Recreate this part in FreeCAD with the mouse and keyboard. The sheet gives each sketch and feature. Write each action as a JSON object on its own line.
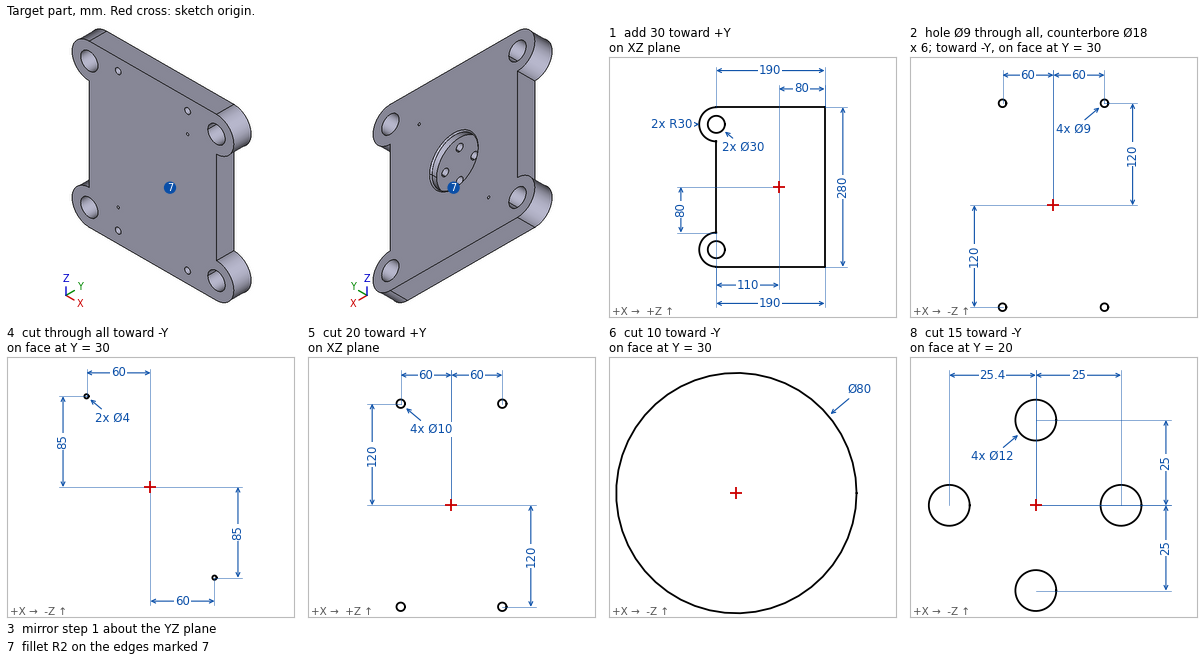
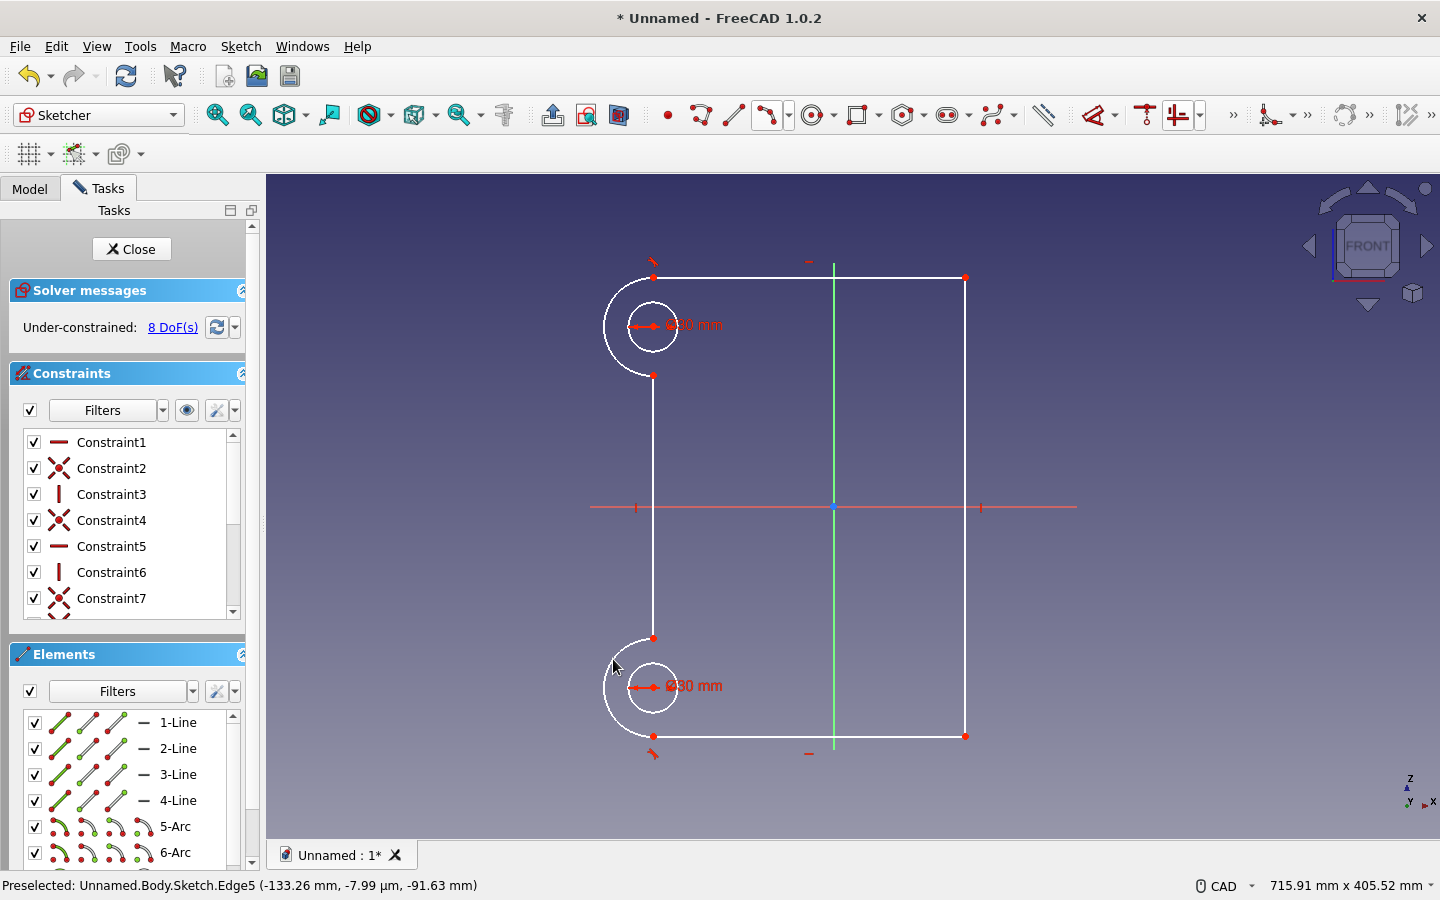
{"action": "left_click", "coordinate": [613, 659]}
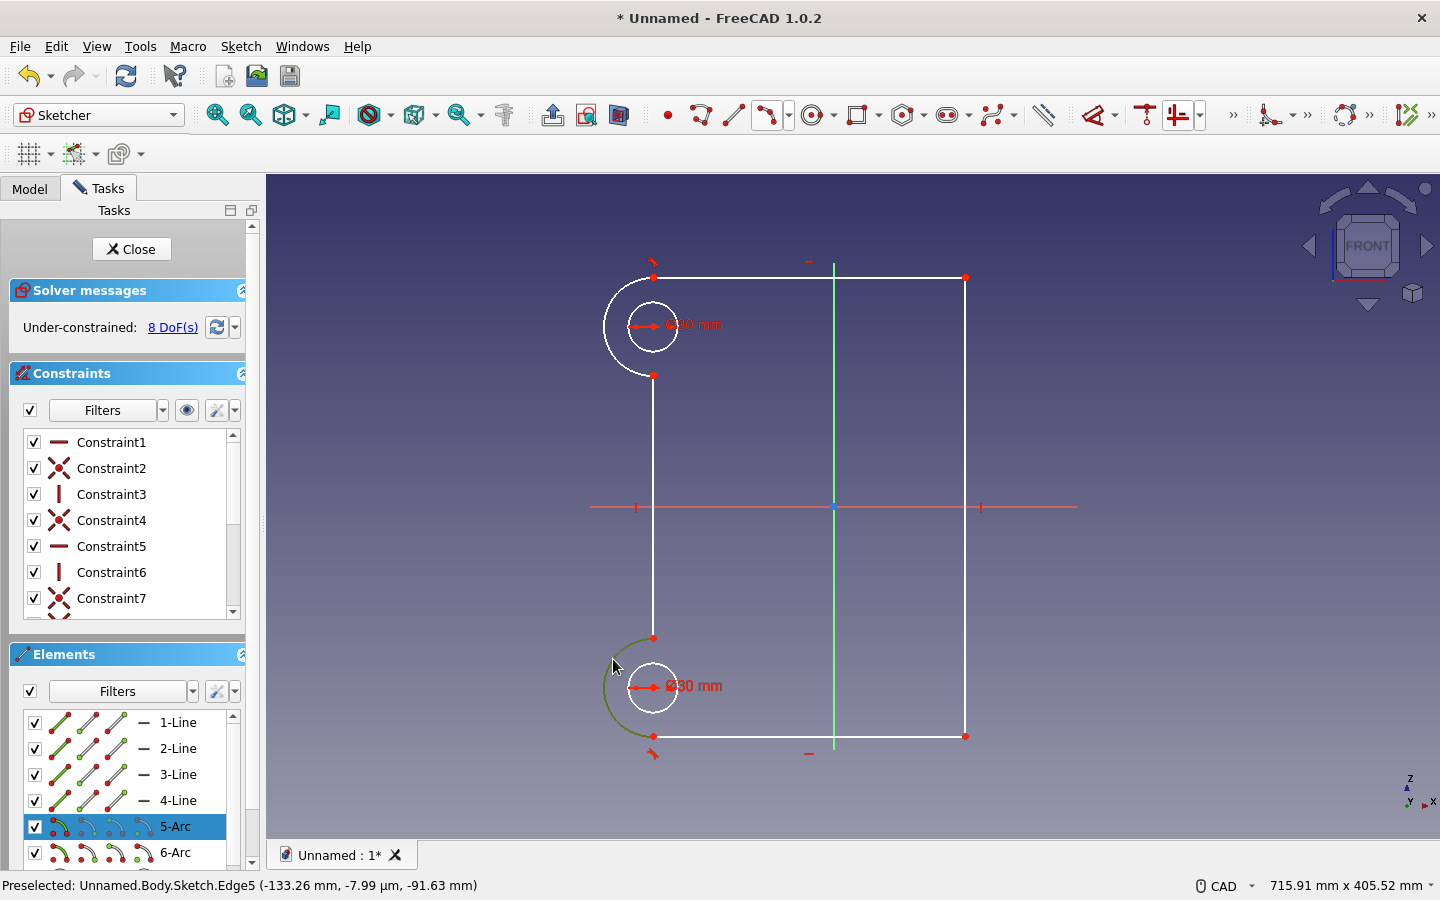
{"action": "left_click", "coordinate": [613, 298]}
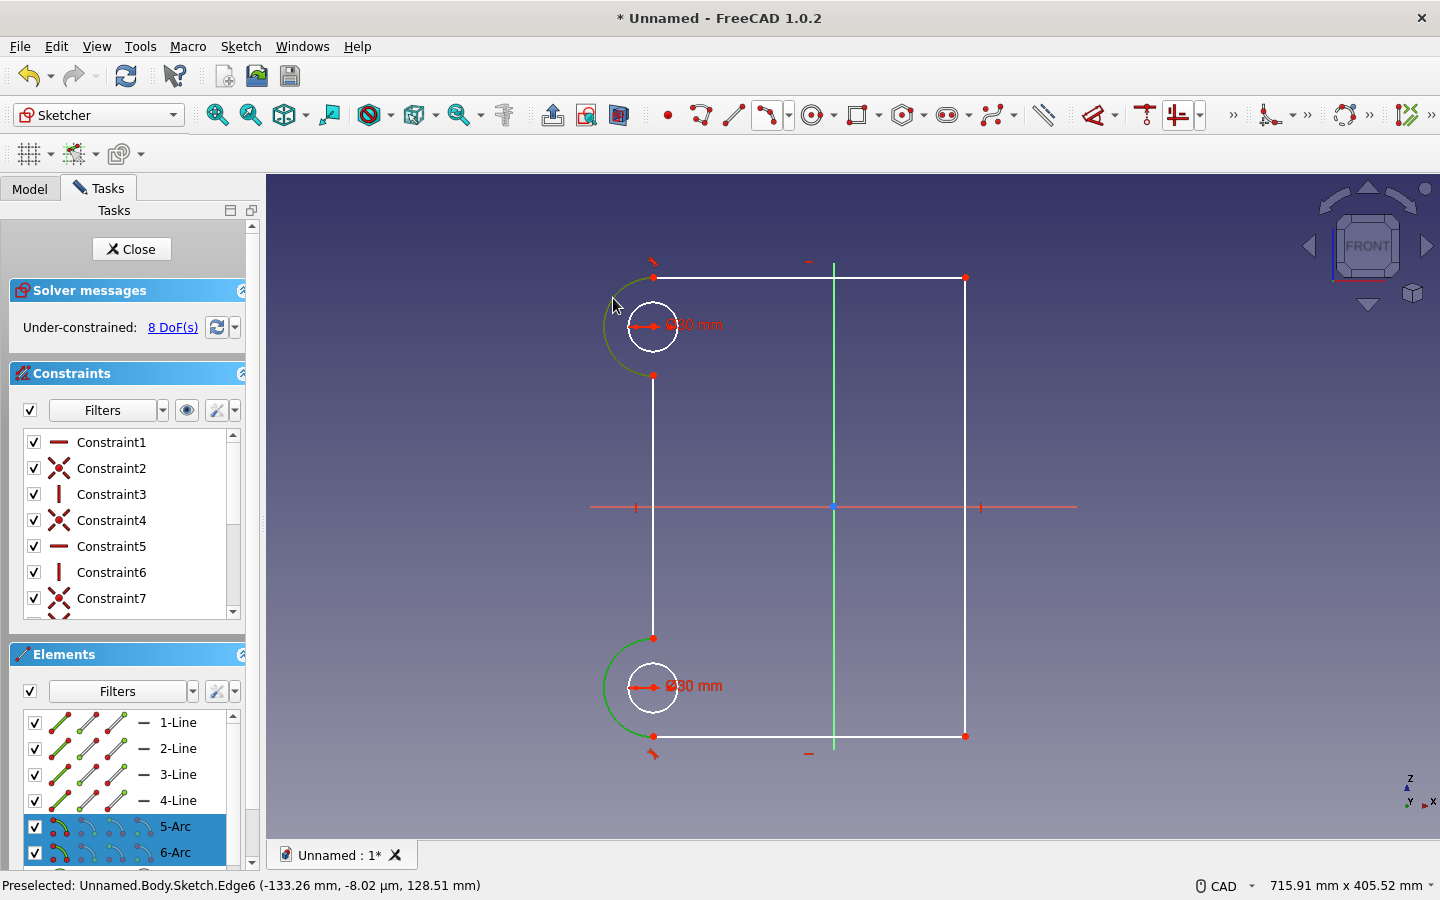
{"action": "key", "text": "e"}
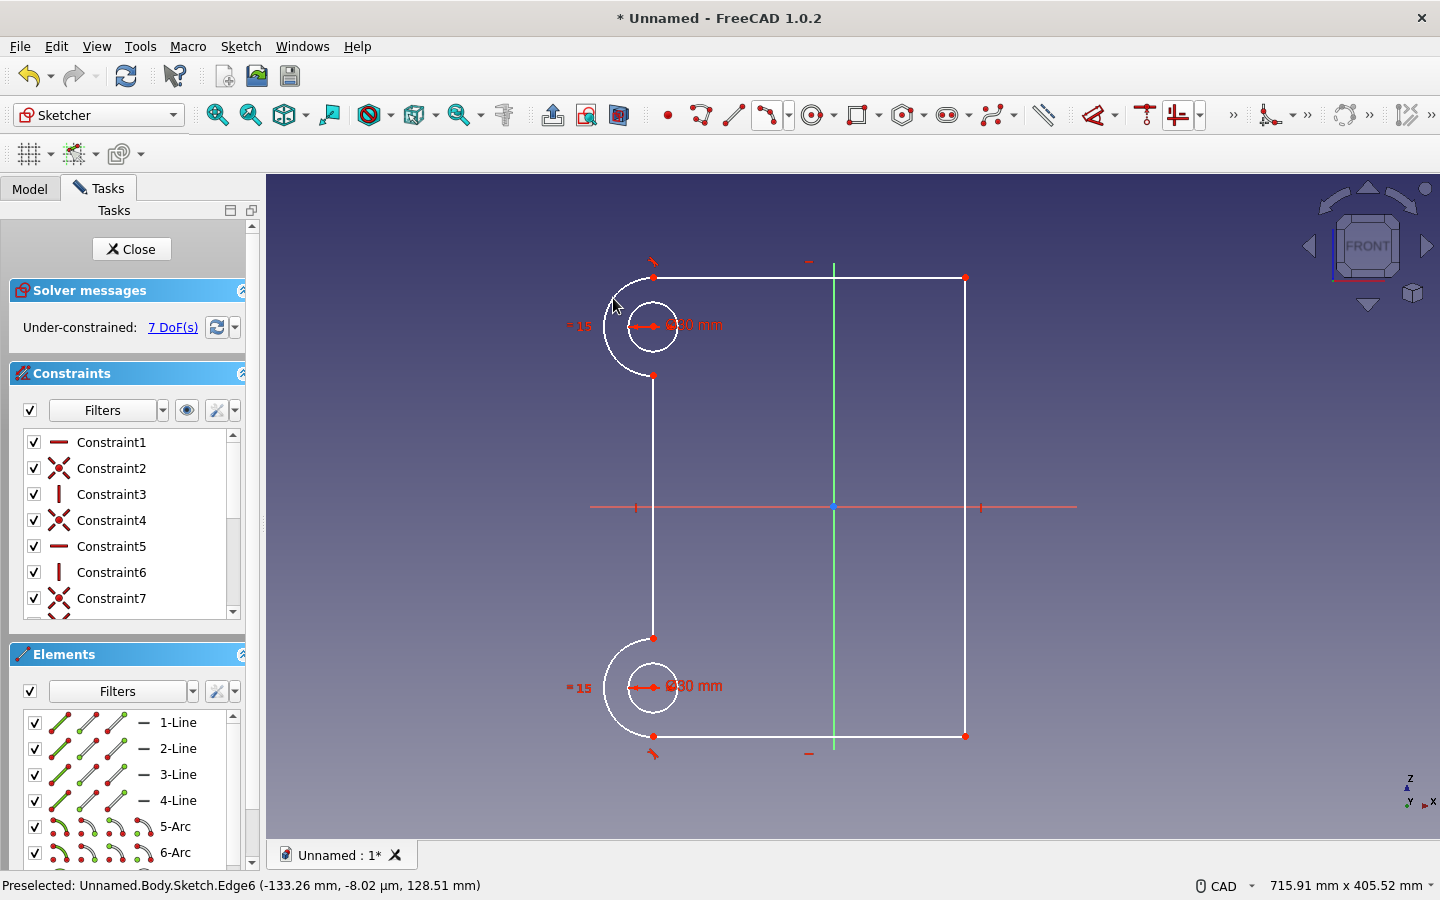
{"action": "left_click", "coordinate": [1092, 116]}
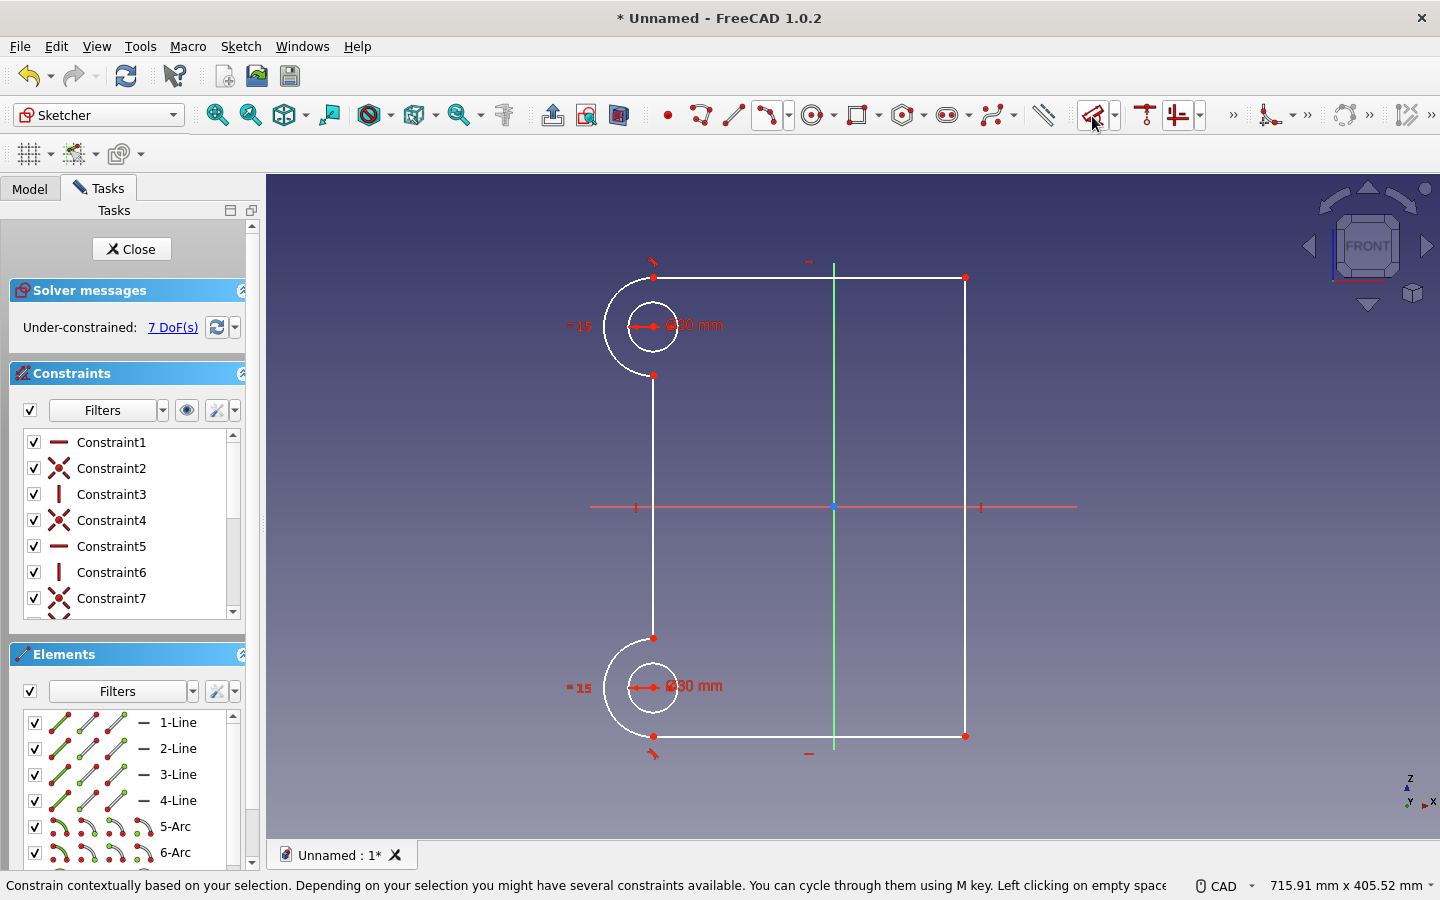
{"action": "left_click", "coordinate": [613, 659]}
{"action": "left_click", "coordinate": [587, 640]}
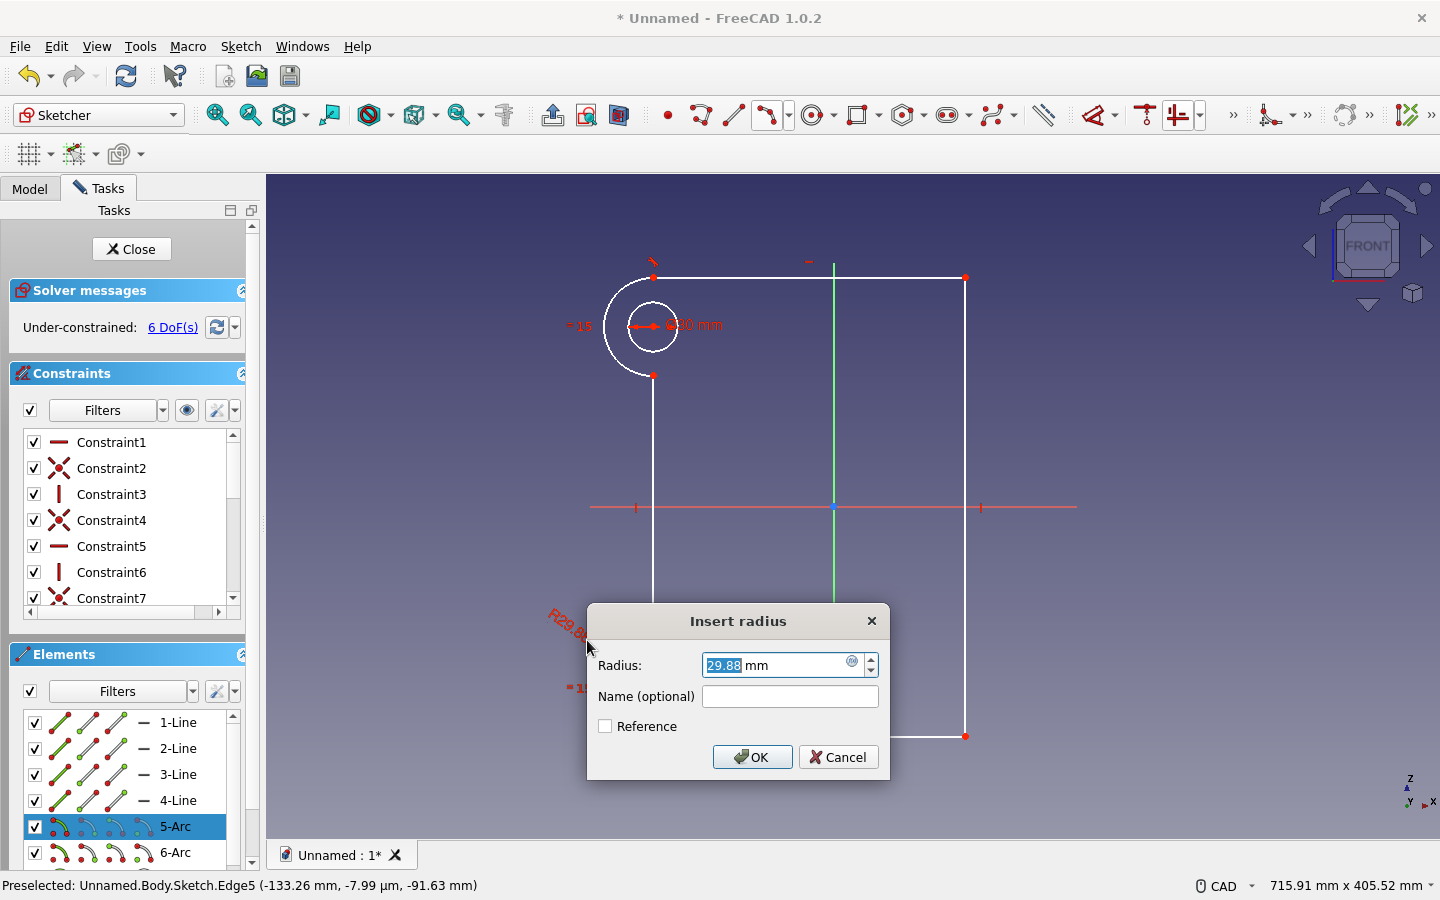
{"action": "type", "text": "30"}
{"action": "key", "text": "Return"}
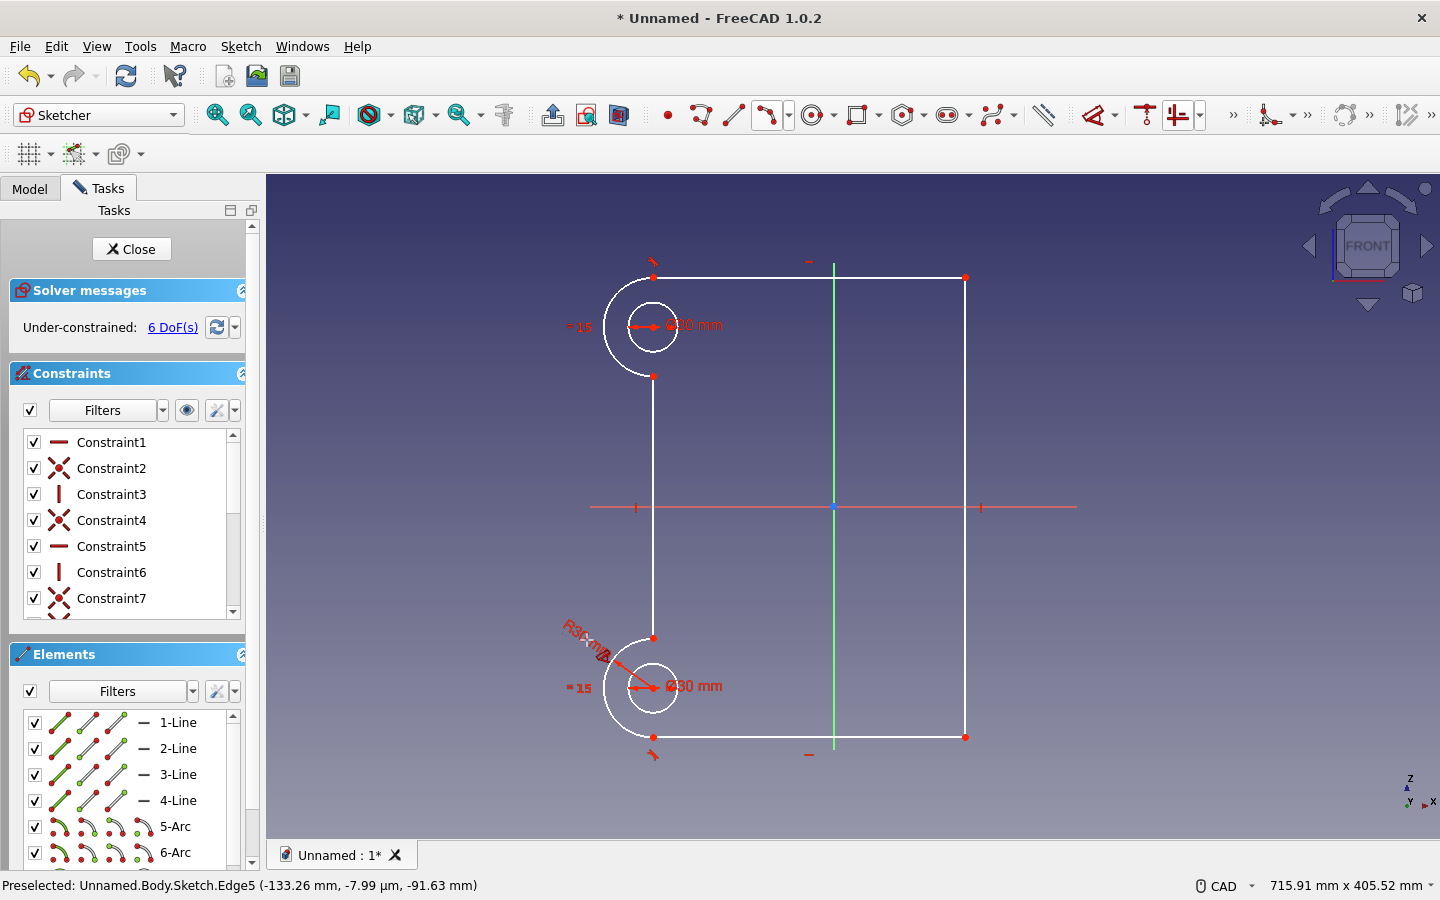
{"action": "left_click", "coordinate": [747, 278]}
{"action": "left_click", "coordinate": [809, 244]}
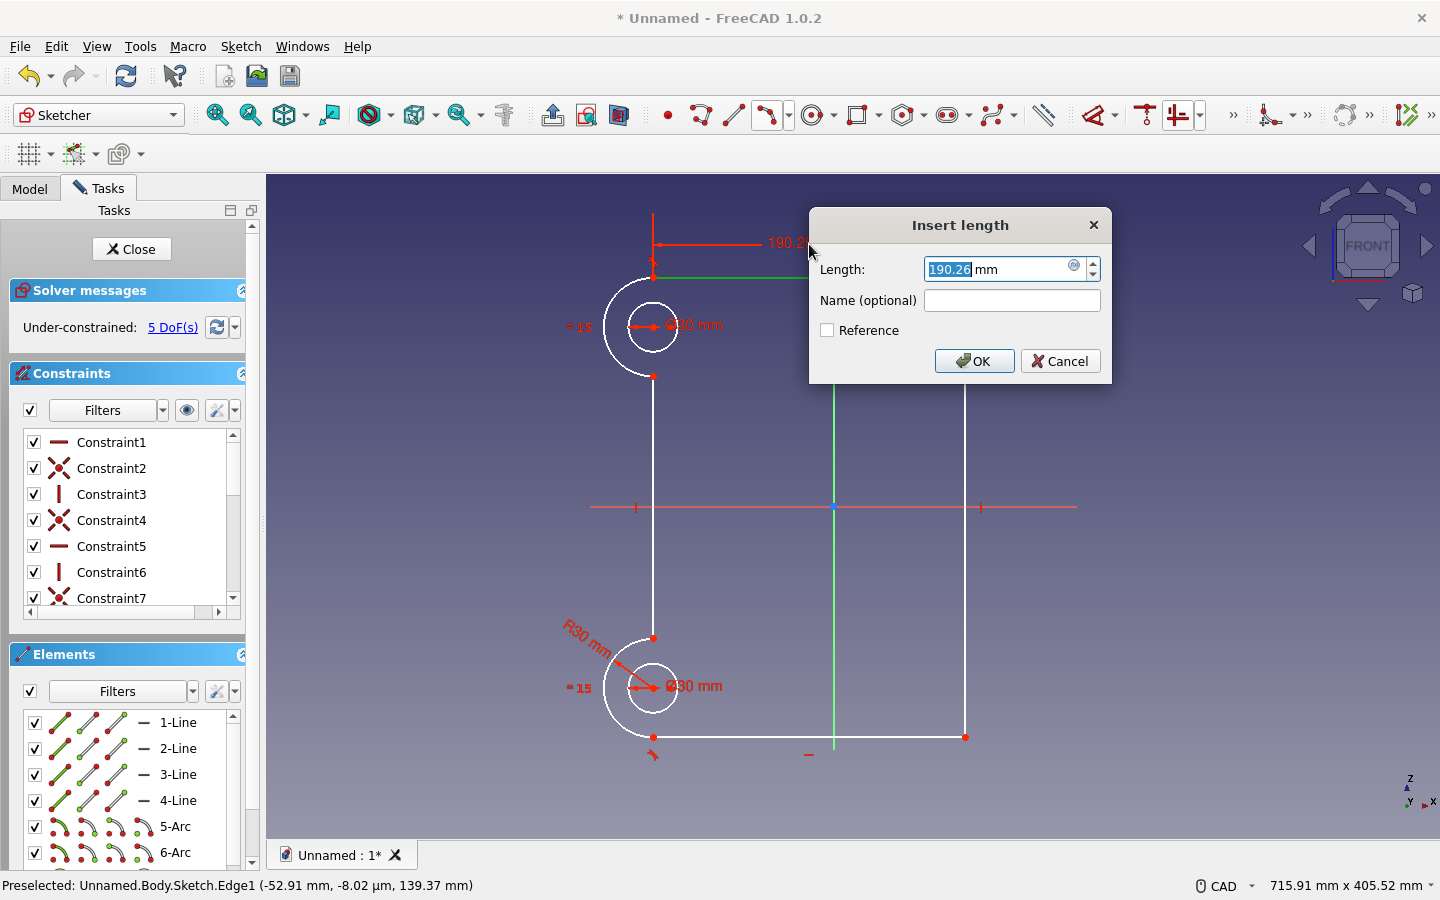
{"action": "type", "text": "190"}
{"action": "key", "text": "Return"}